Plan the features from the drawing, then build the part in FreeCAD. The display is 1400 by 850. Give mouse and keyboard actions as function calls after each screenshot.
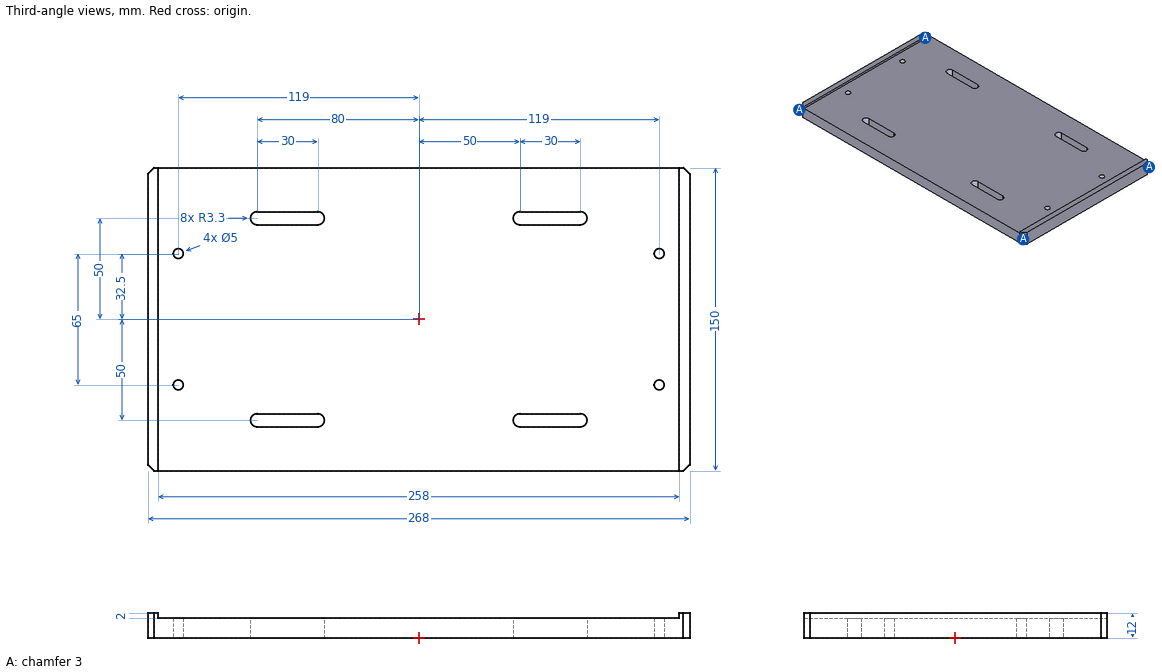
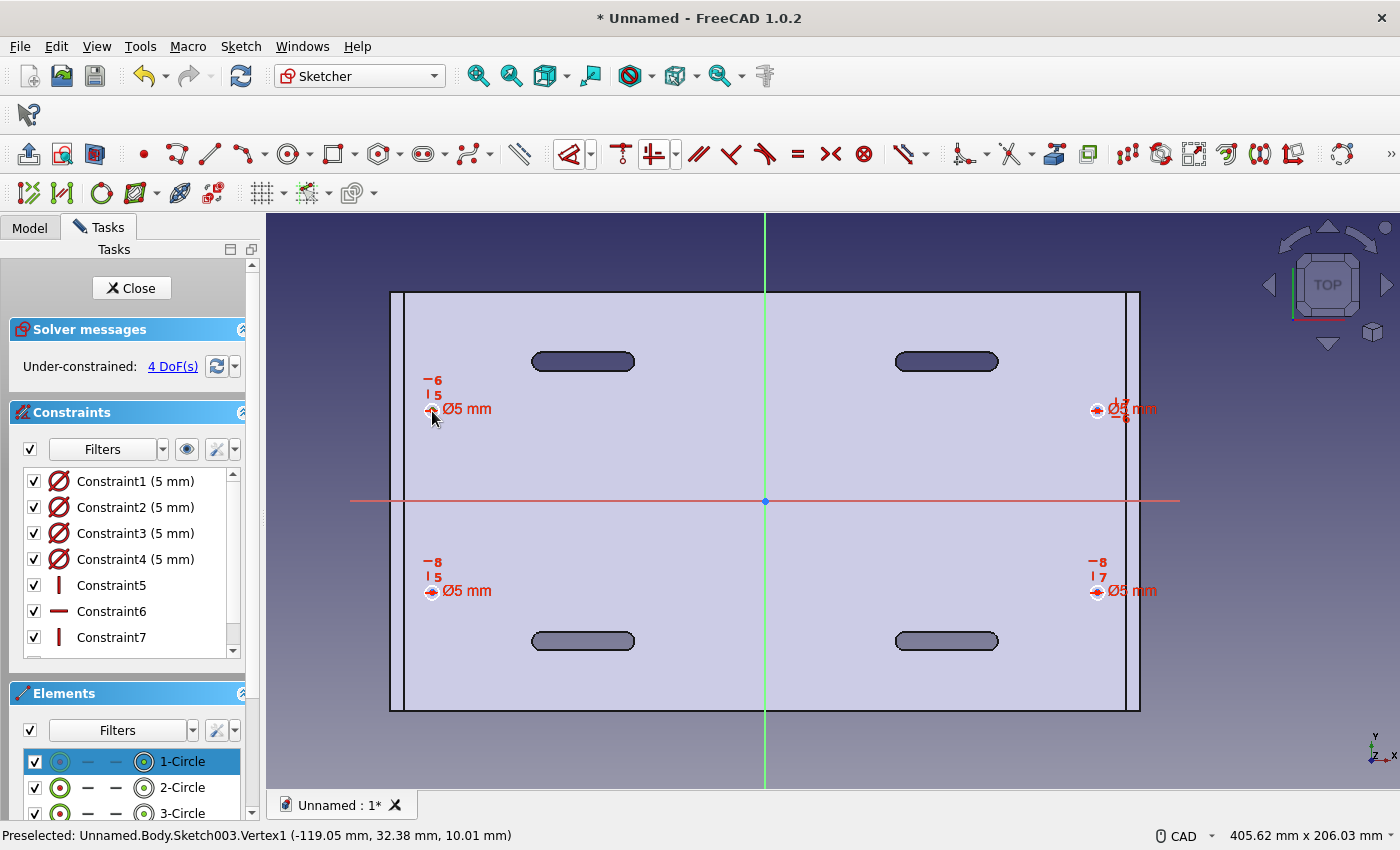
click(590, 154)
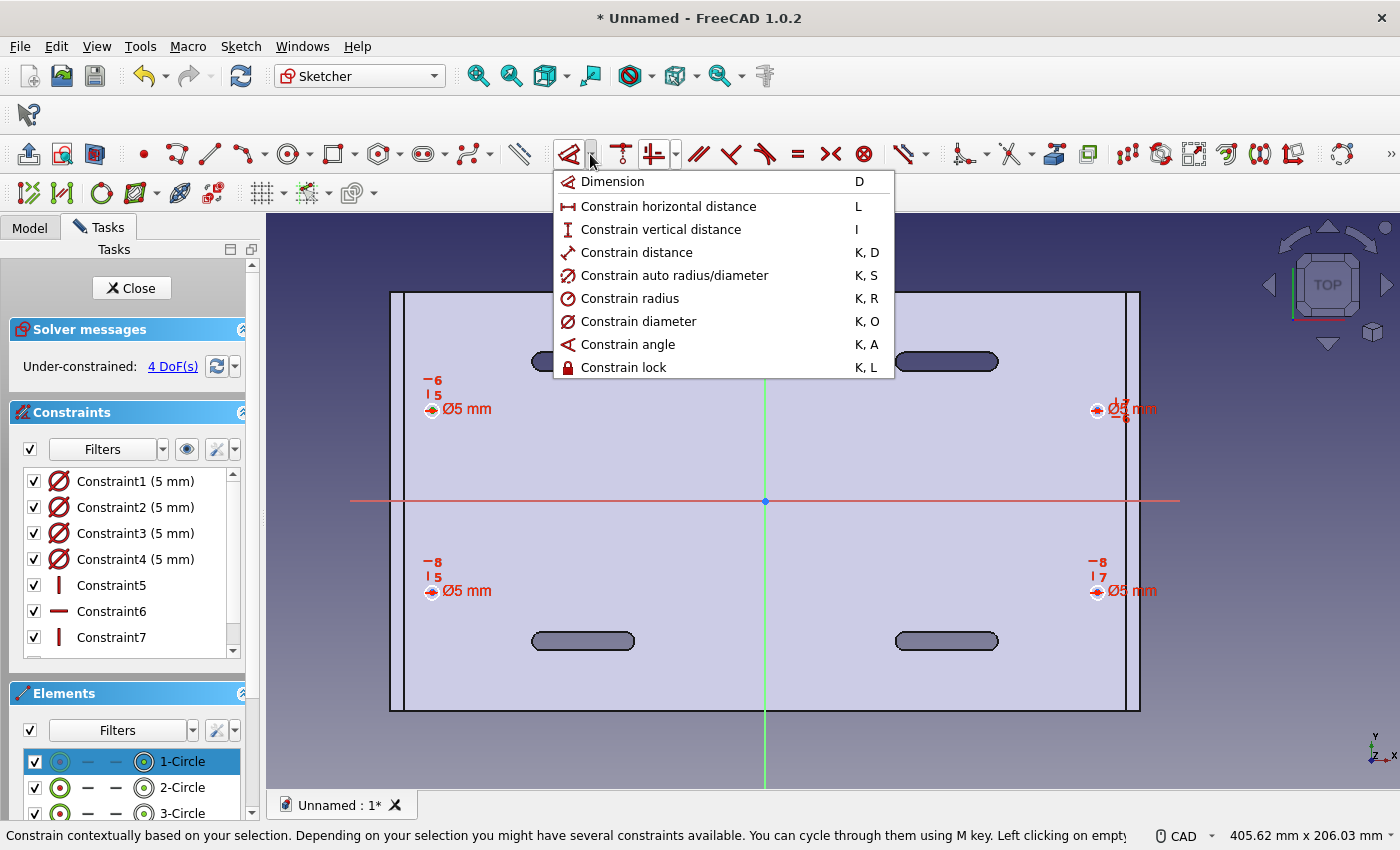
click(724, 206)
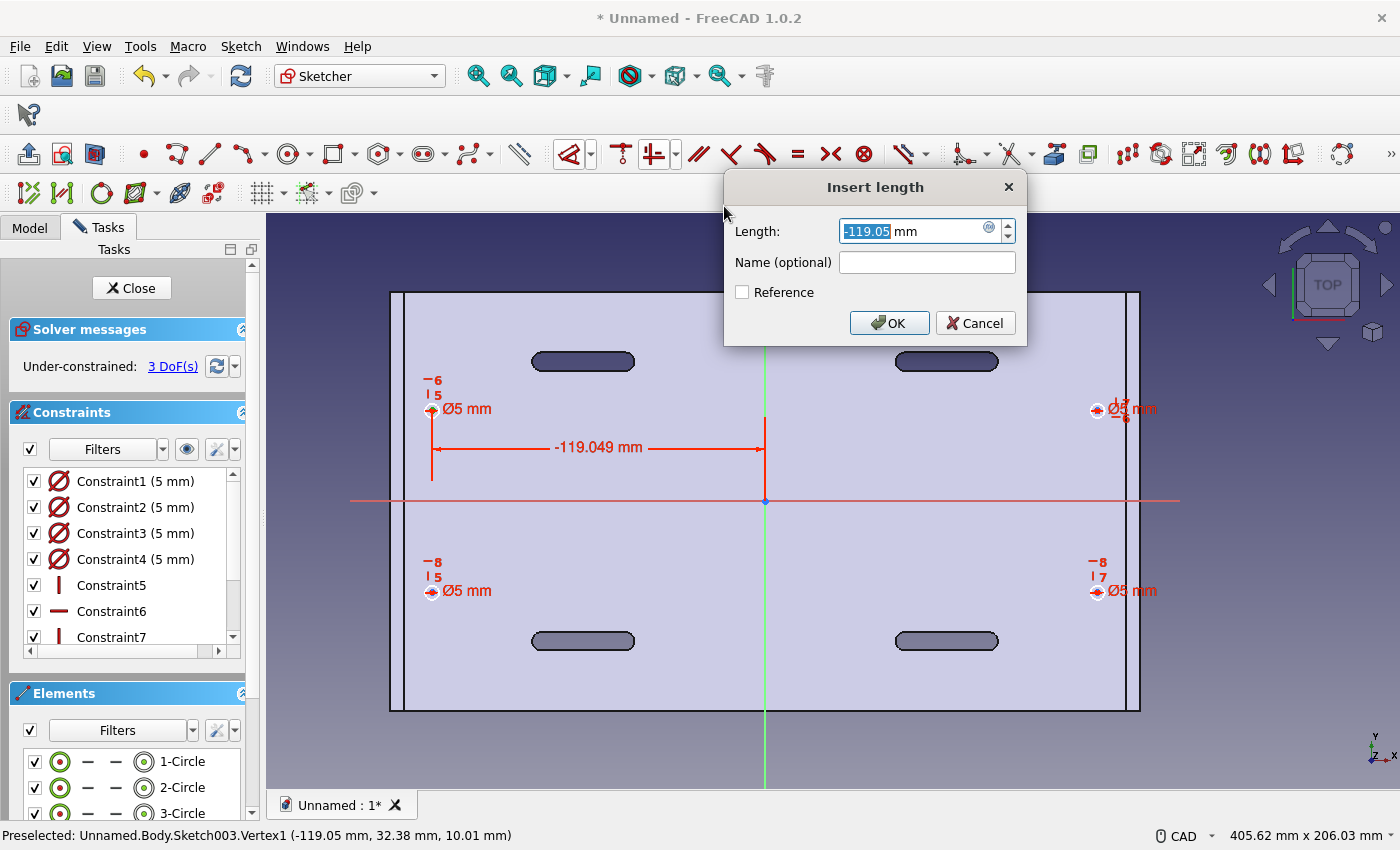
text(-119)
key(Return)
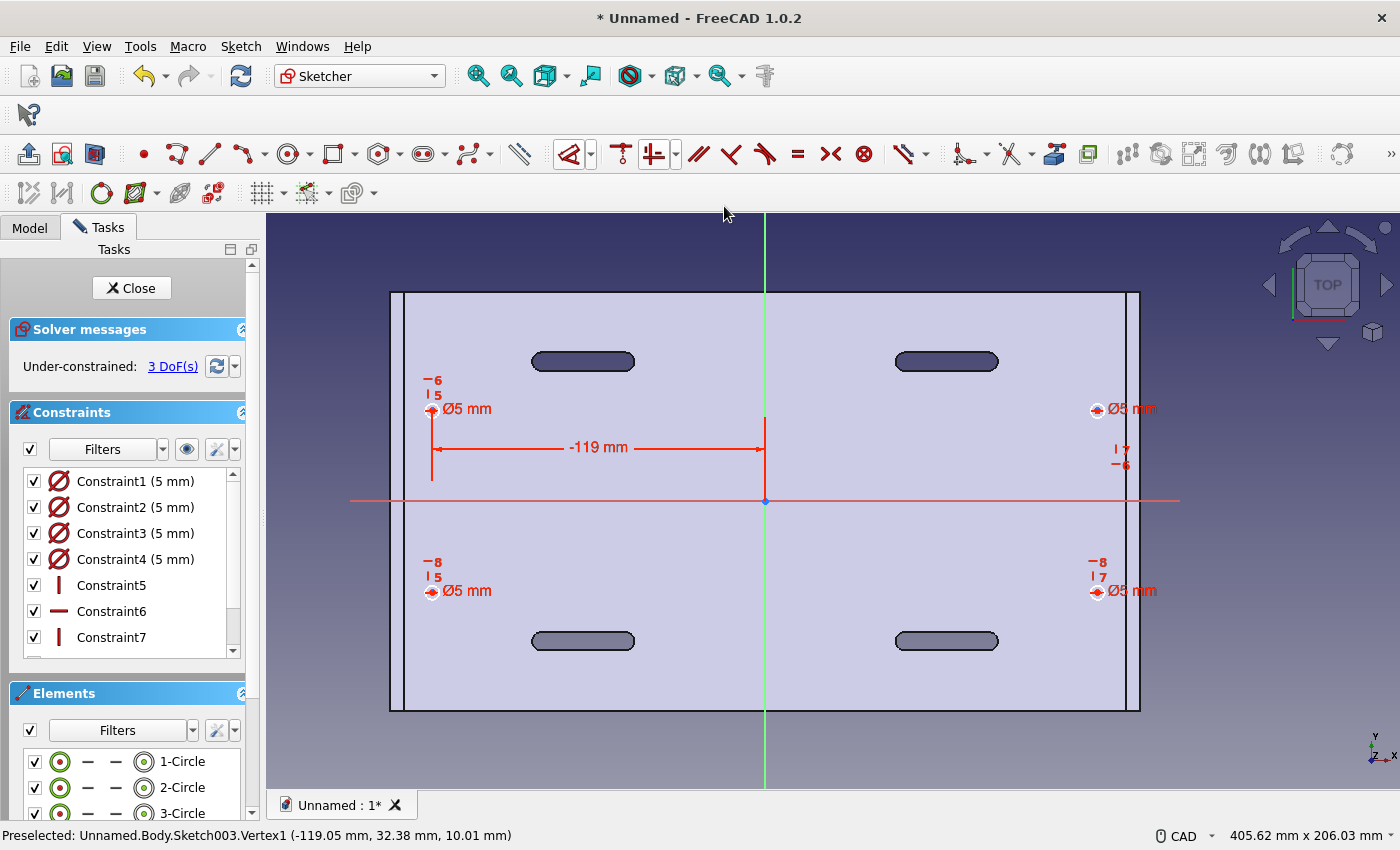
click(1098, 411)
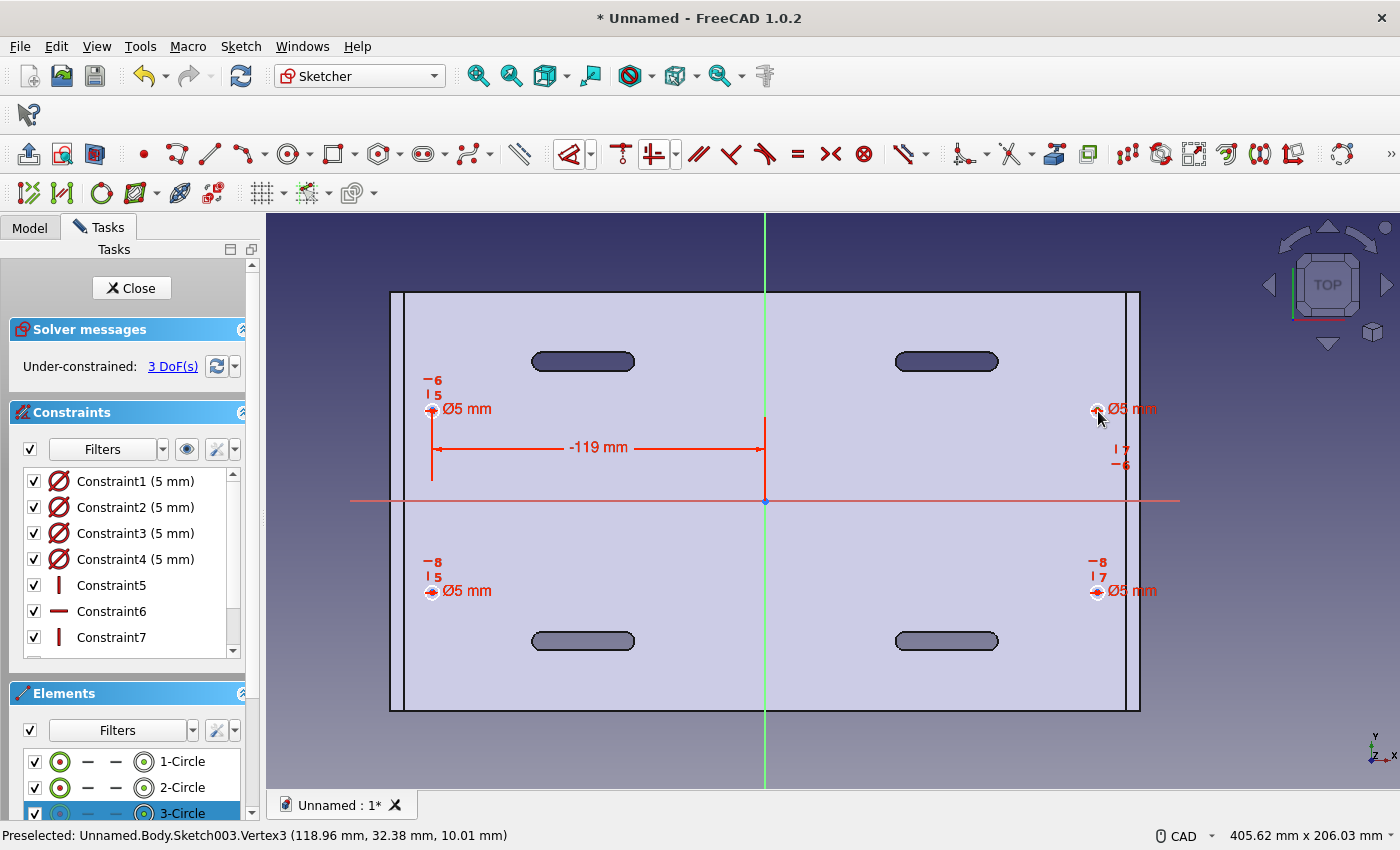
key(l)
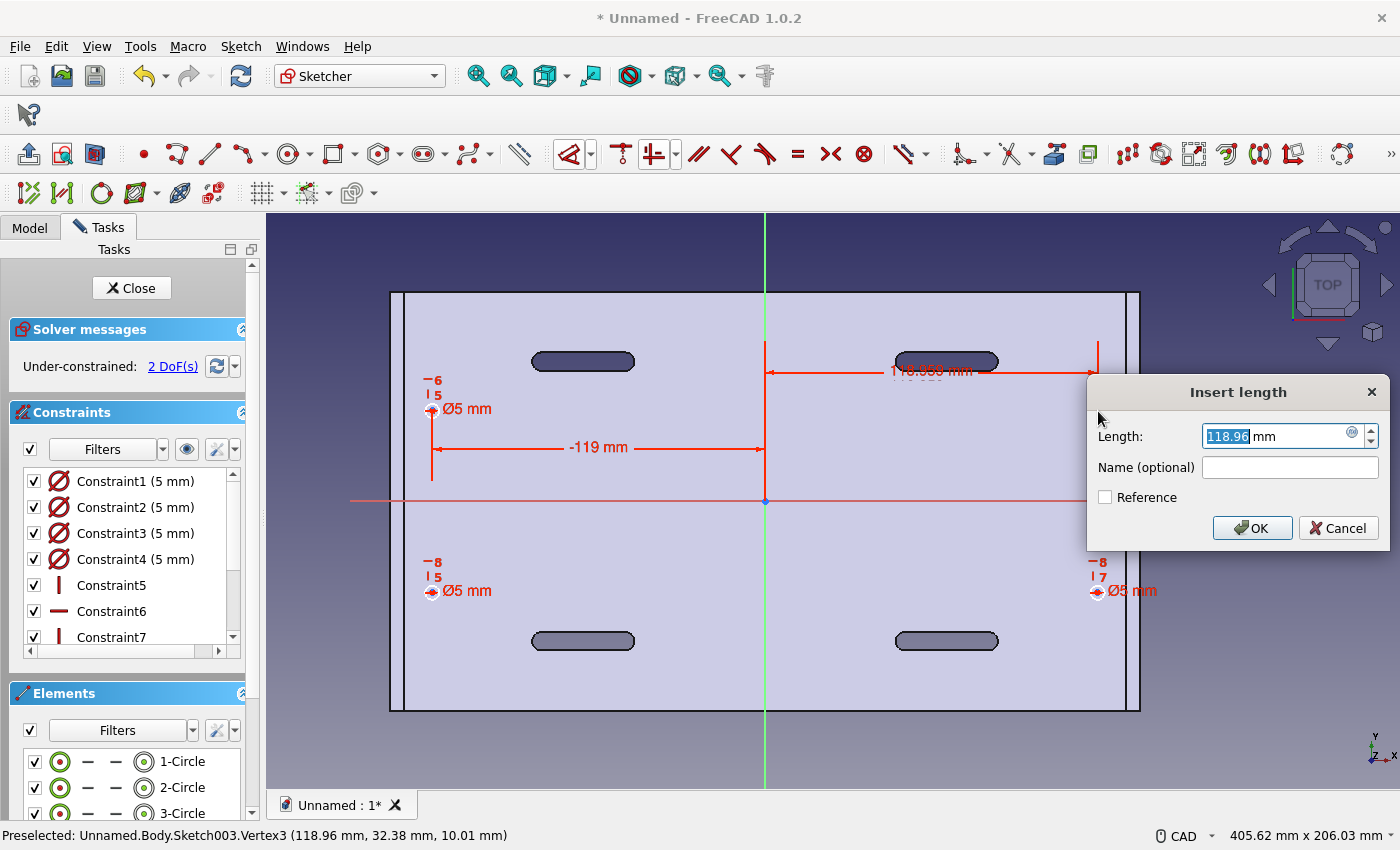
text(119)
key(Return)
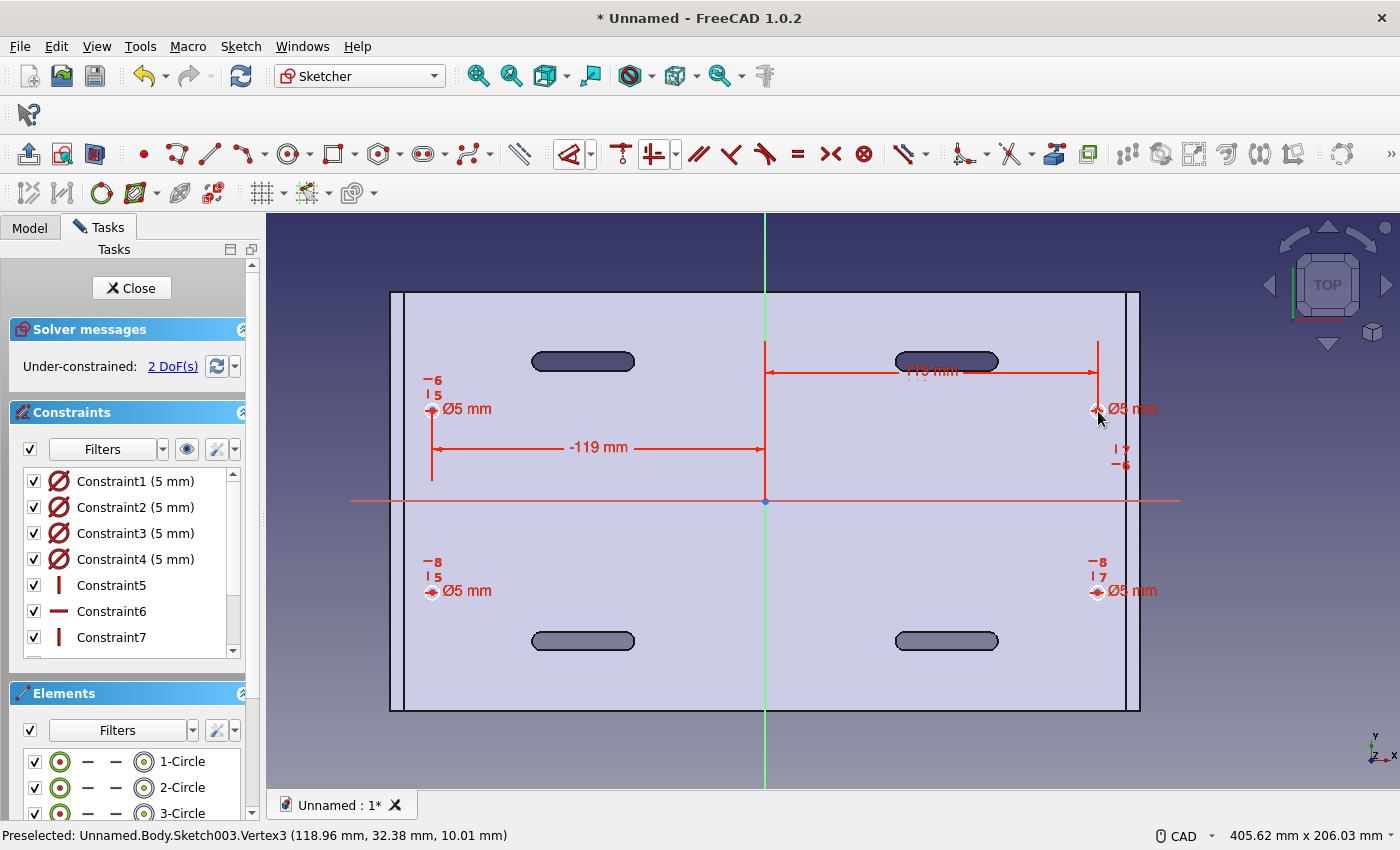
click(432, 411)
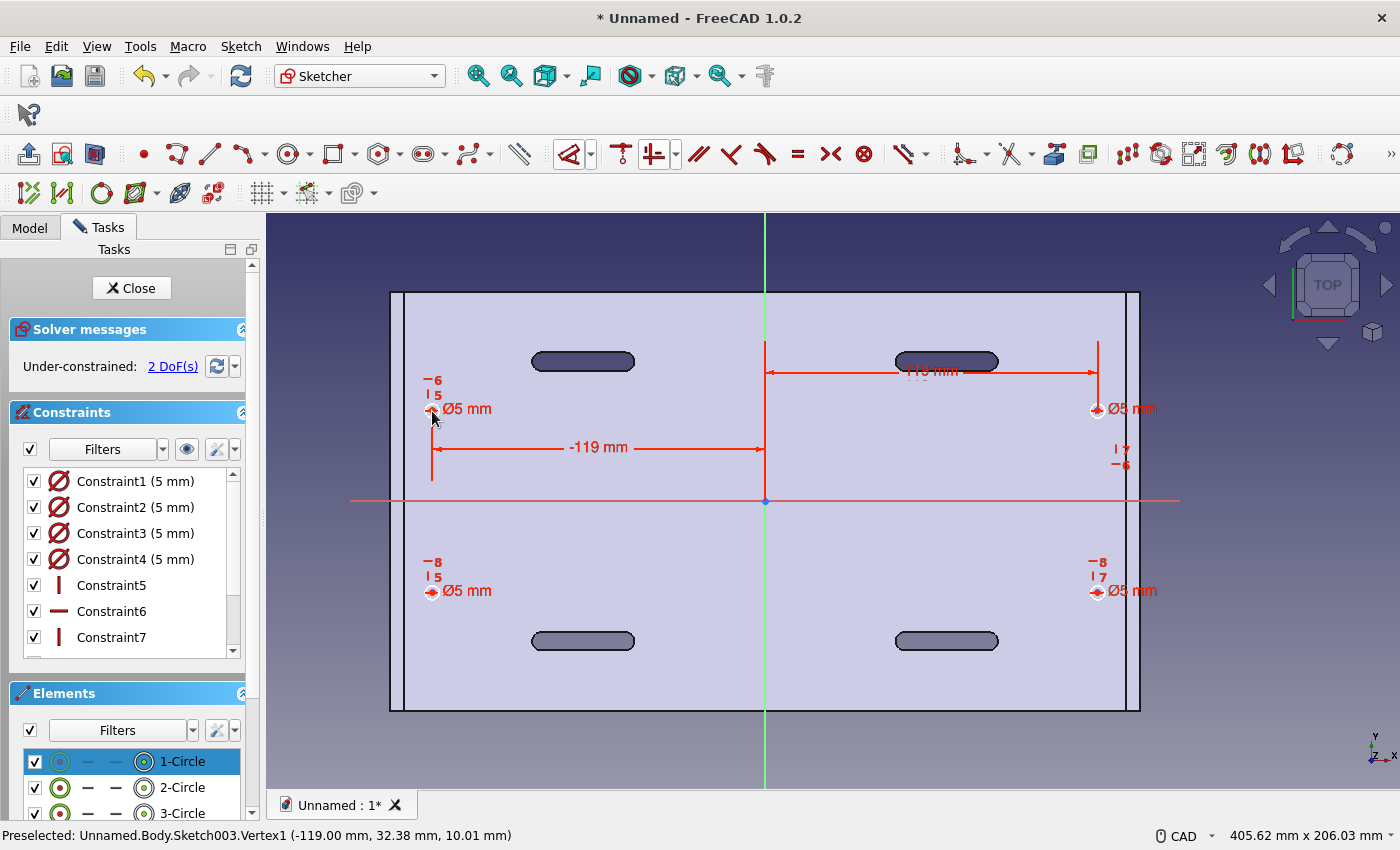
click(432, 593)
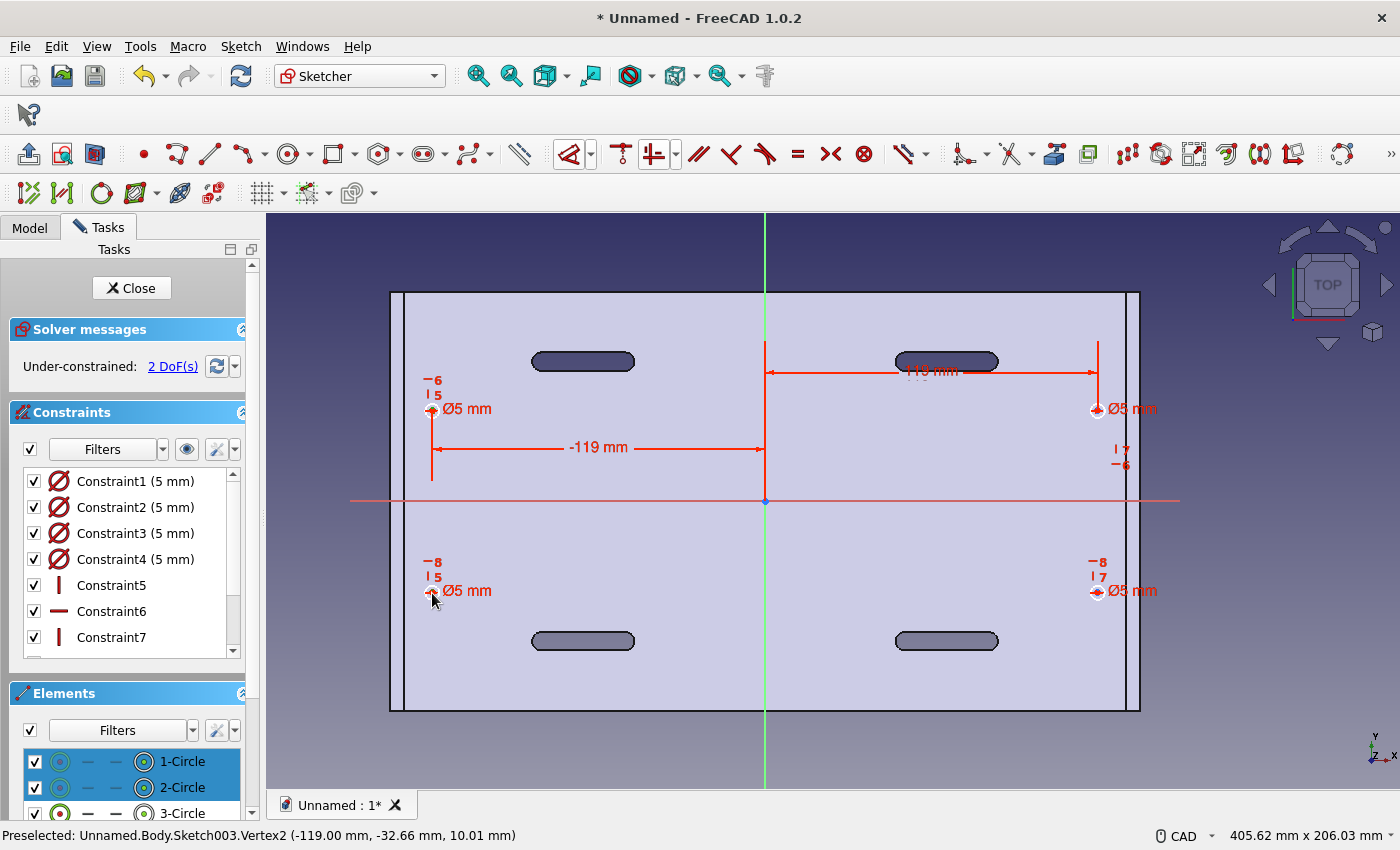
click(590, 154)